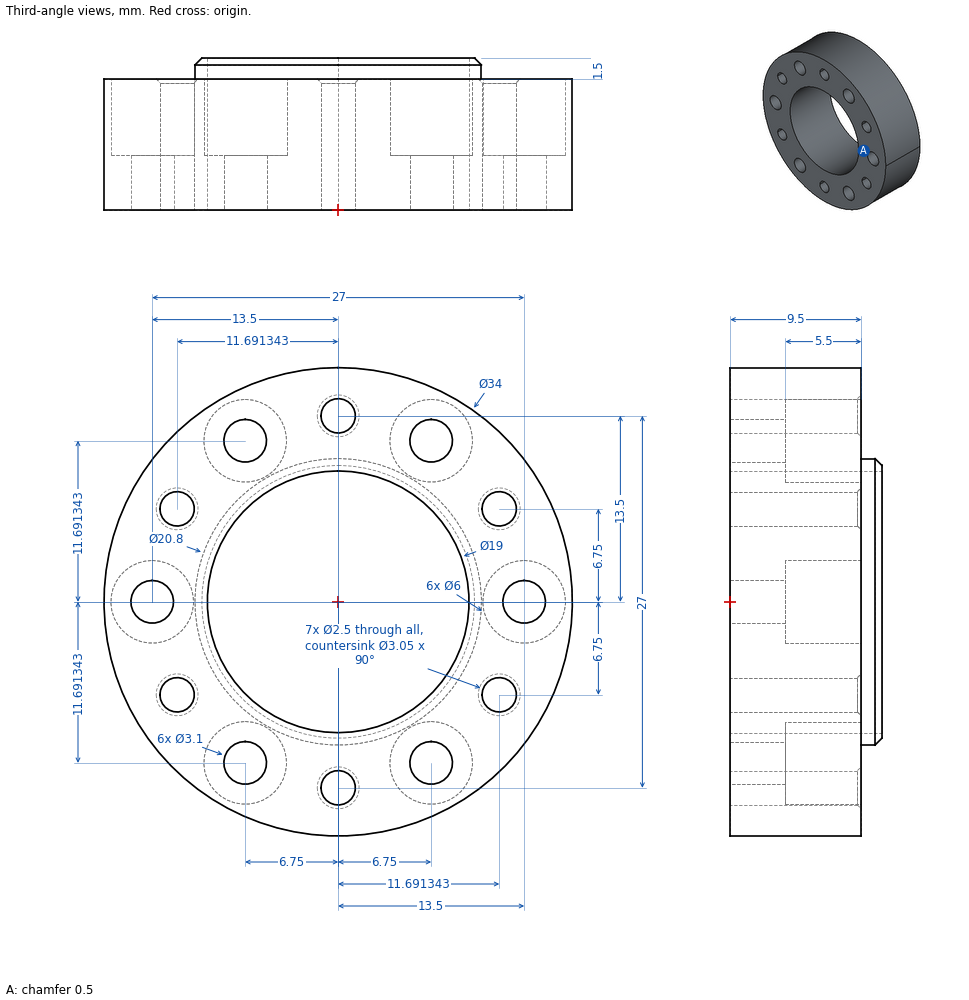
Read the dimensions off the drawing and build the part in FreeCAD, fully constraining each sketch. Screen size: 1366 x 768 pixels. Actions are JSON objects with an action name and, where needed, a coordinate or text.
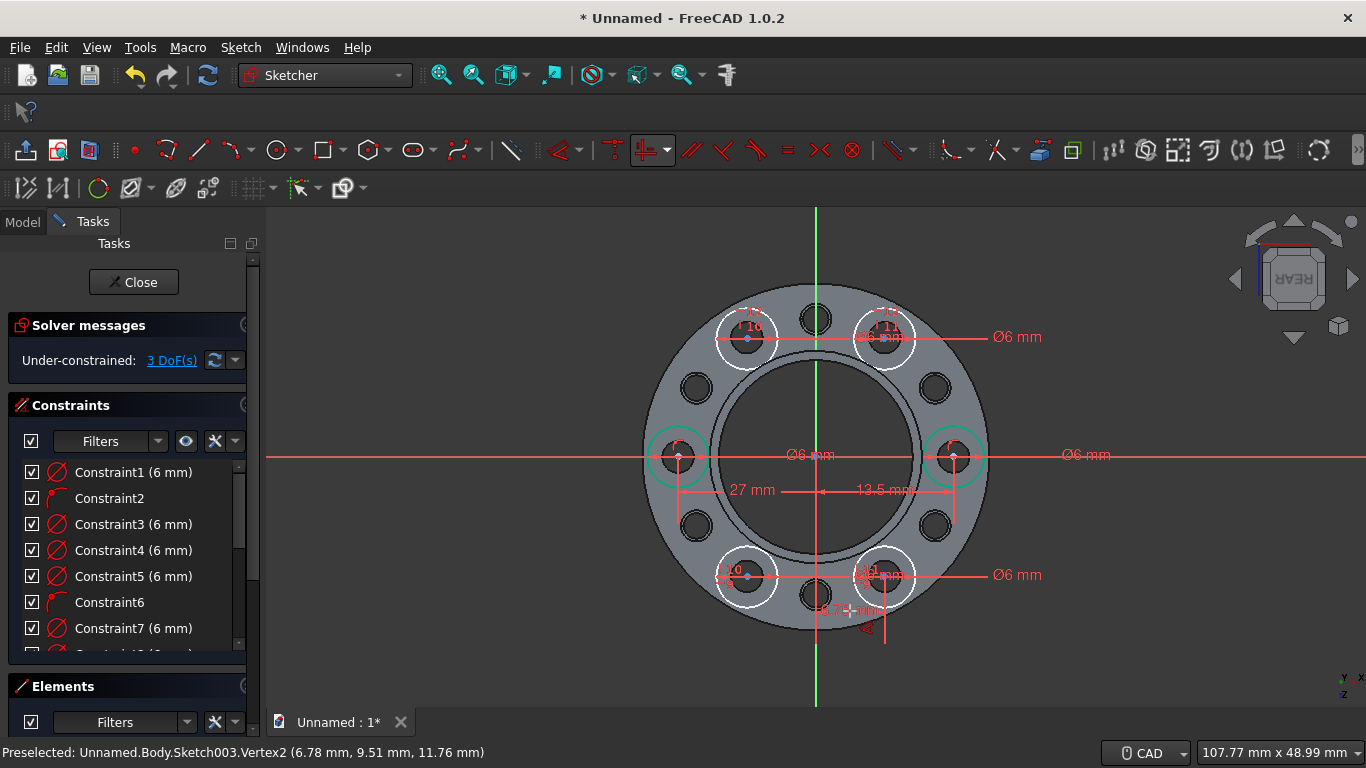
{"action": "left_click", "coordinate": [747, 577]}
{"action": "left_click", "coordinate": [781, 423]}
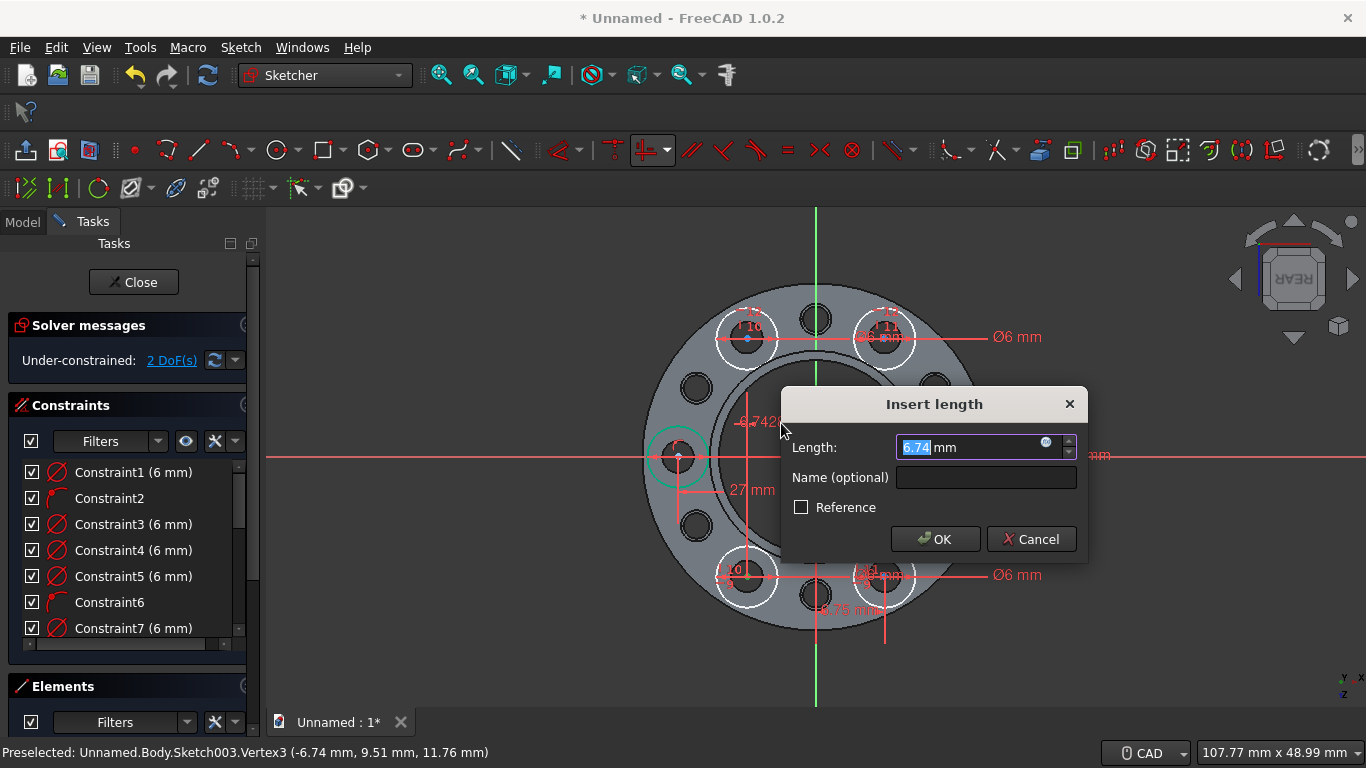
{"action": "type", "text": "6.75"}
{"action": "key", "text": "Return"}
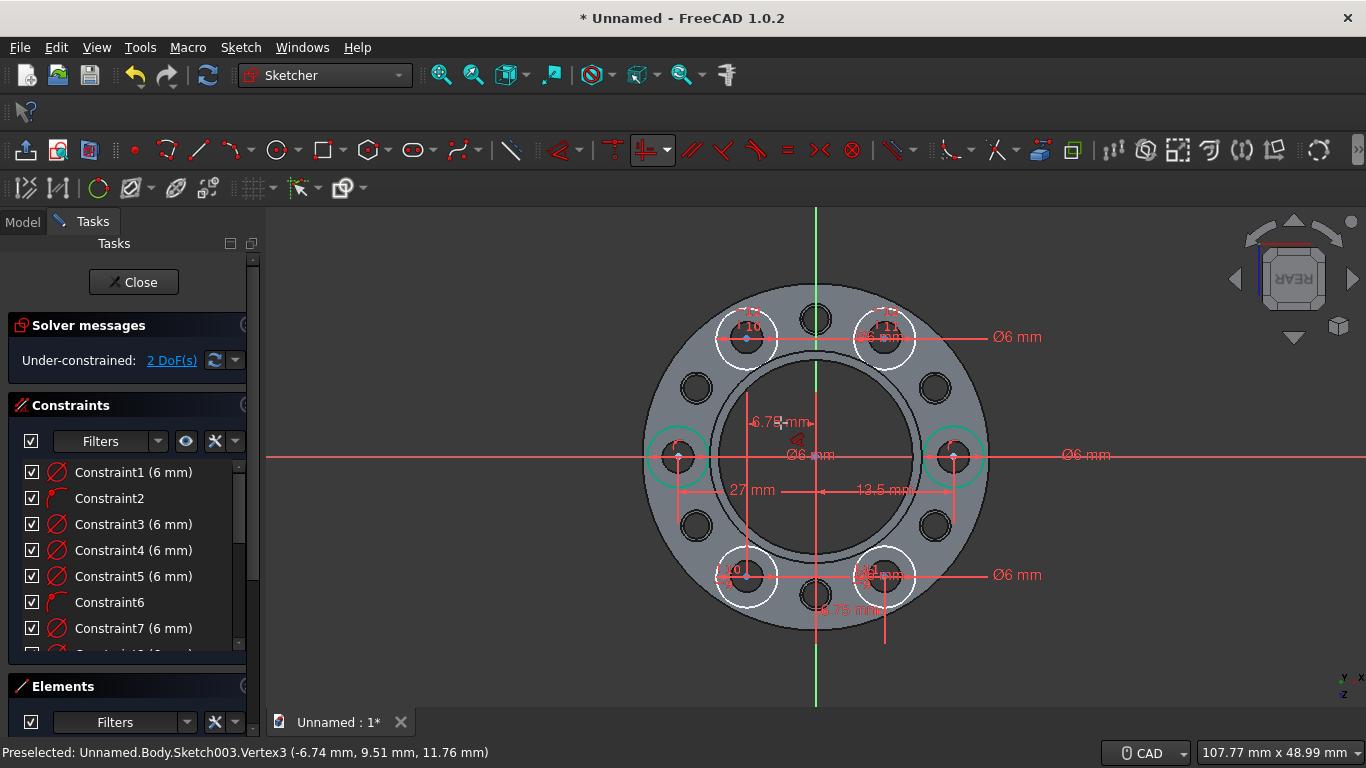
{"action": "left_click", "coordinate": [885, 577]}
{"action": "left_click", "coordinate": [919, 517]}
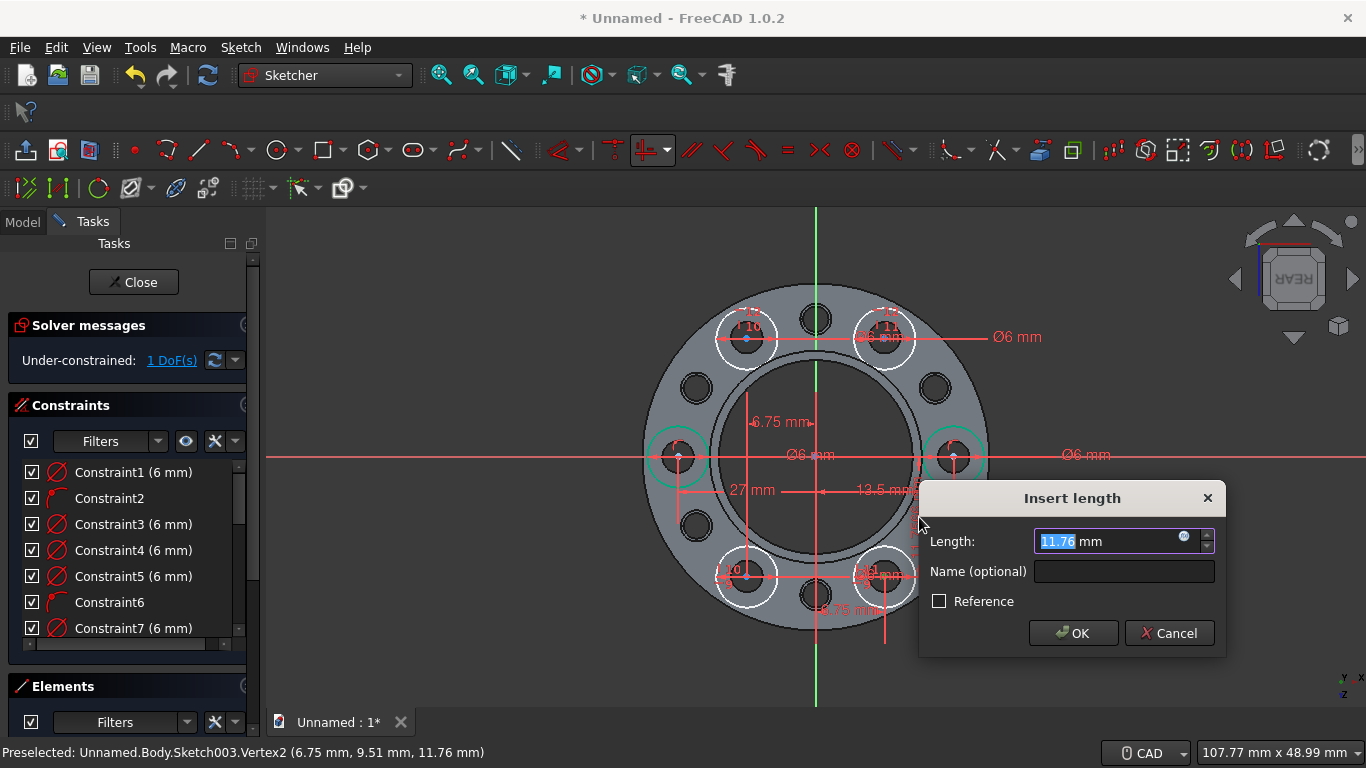
{"action": "type", "text": "11.691343"}
{"action": "key", "text": "Return"}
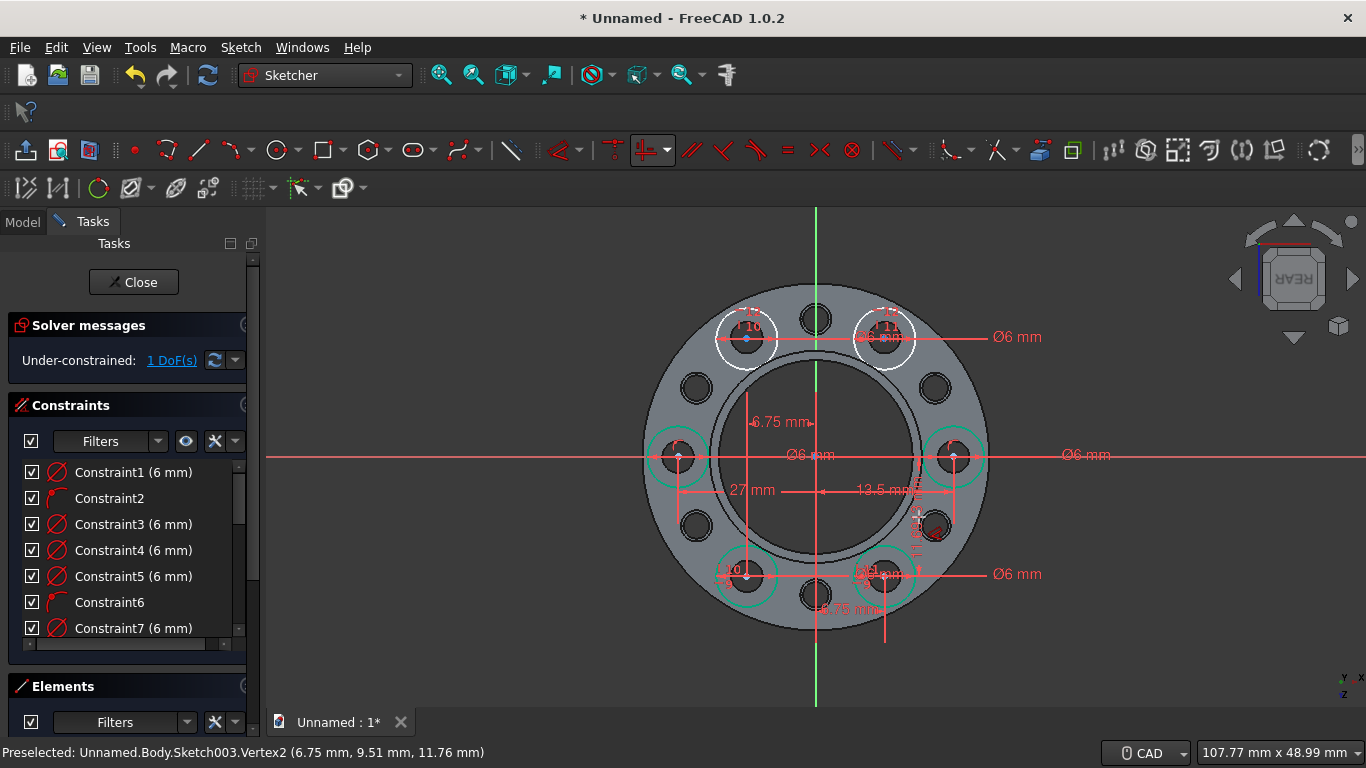
{"action": "left_click", "coordinate": [747, 339]}
{"action": "left_click", "coordinate": [713, 398]}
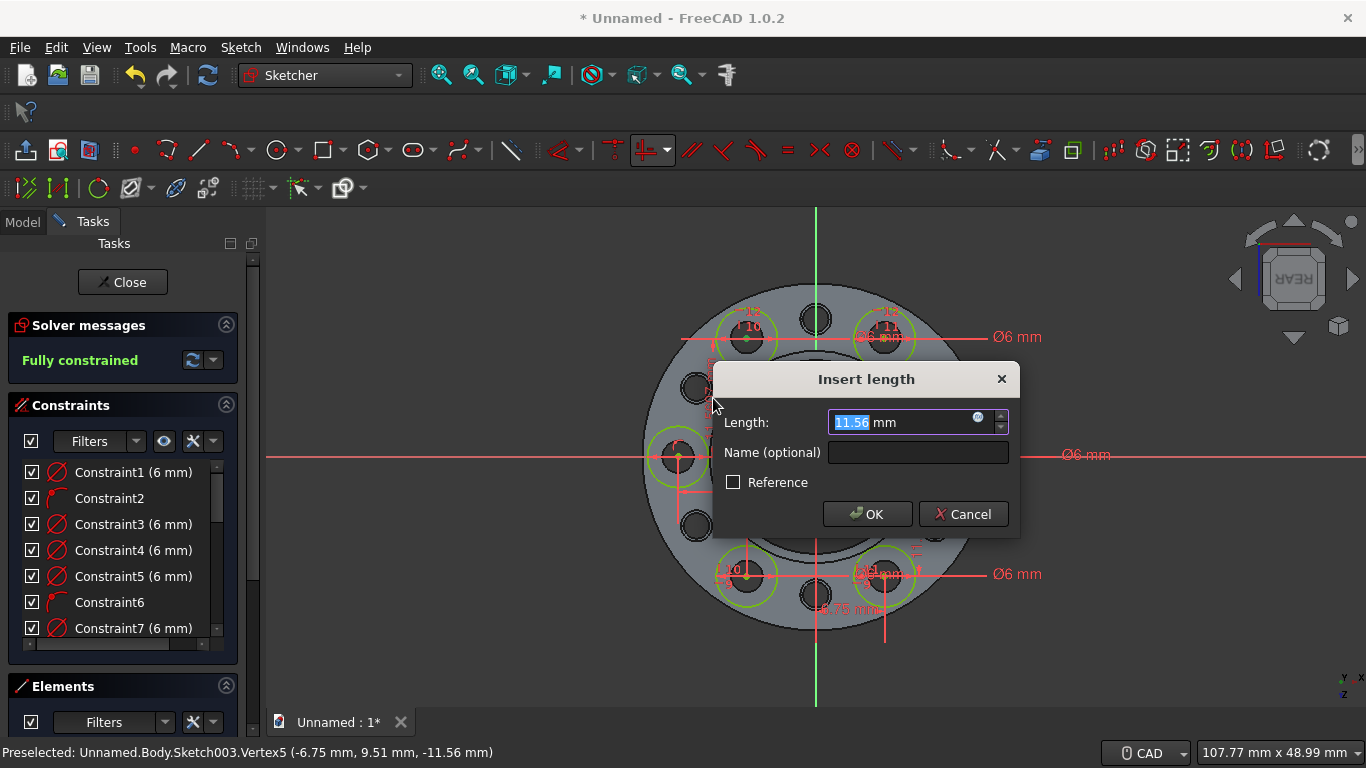
{"action": "type", "text": "11.691343"}
{"action": "key", "text": "Return"}
{"action": "key", "text": "Escape"}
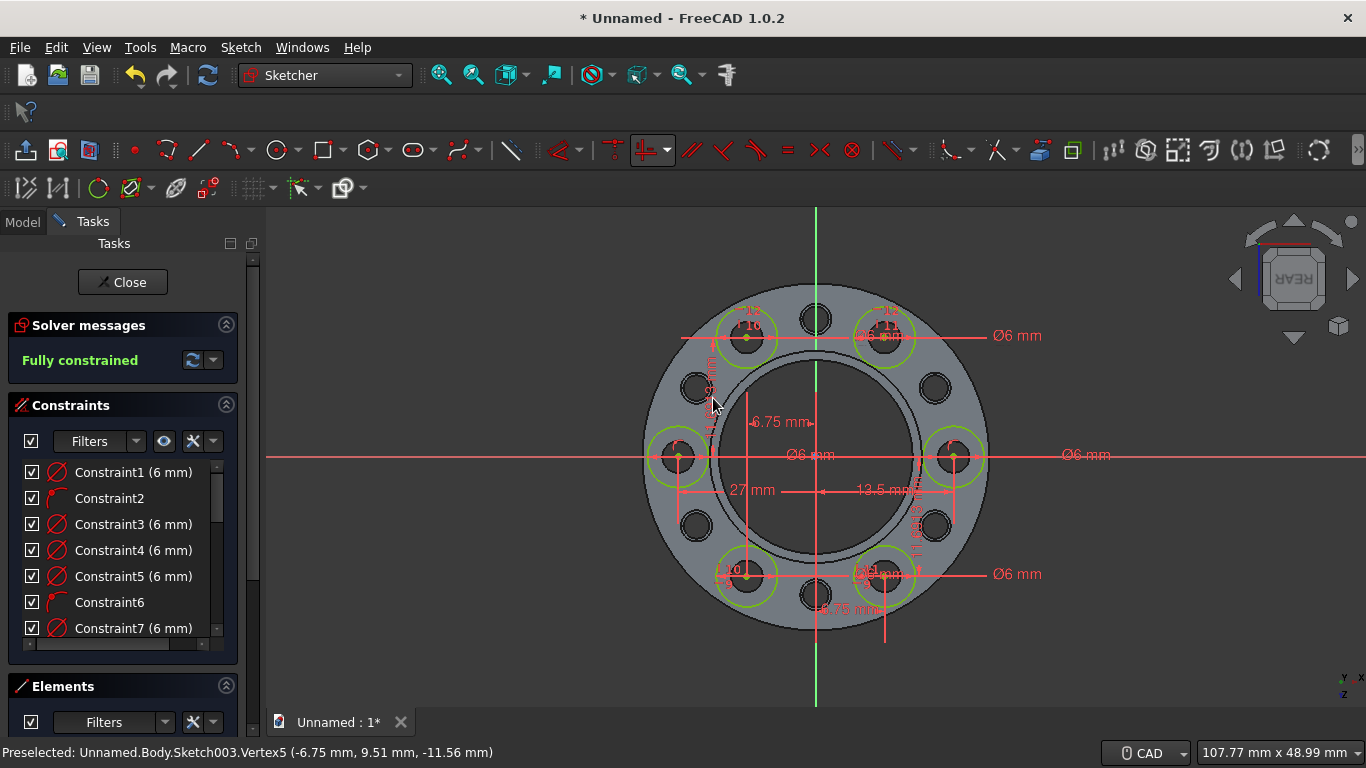
{"action": "left_click", "coordinate": [123, 282]}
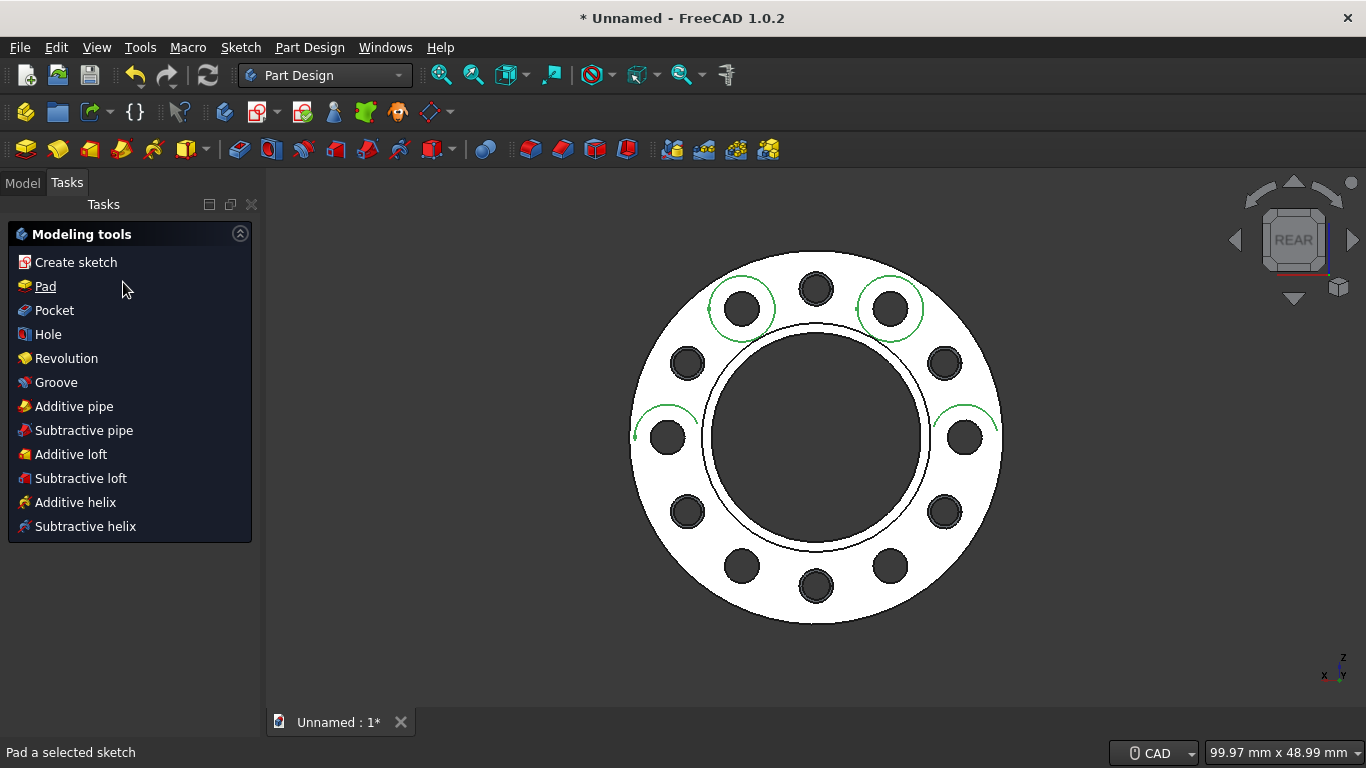
{"action": "left_click", "coordinate": [240, 150]}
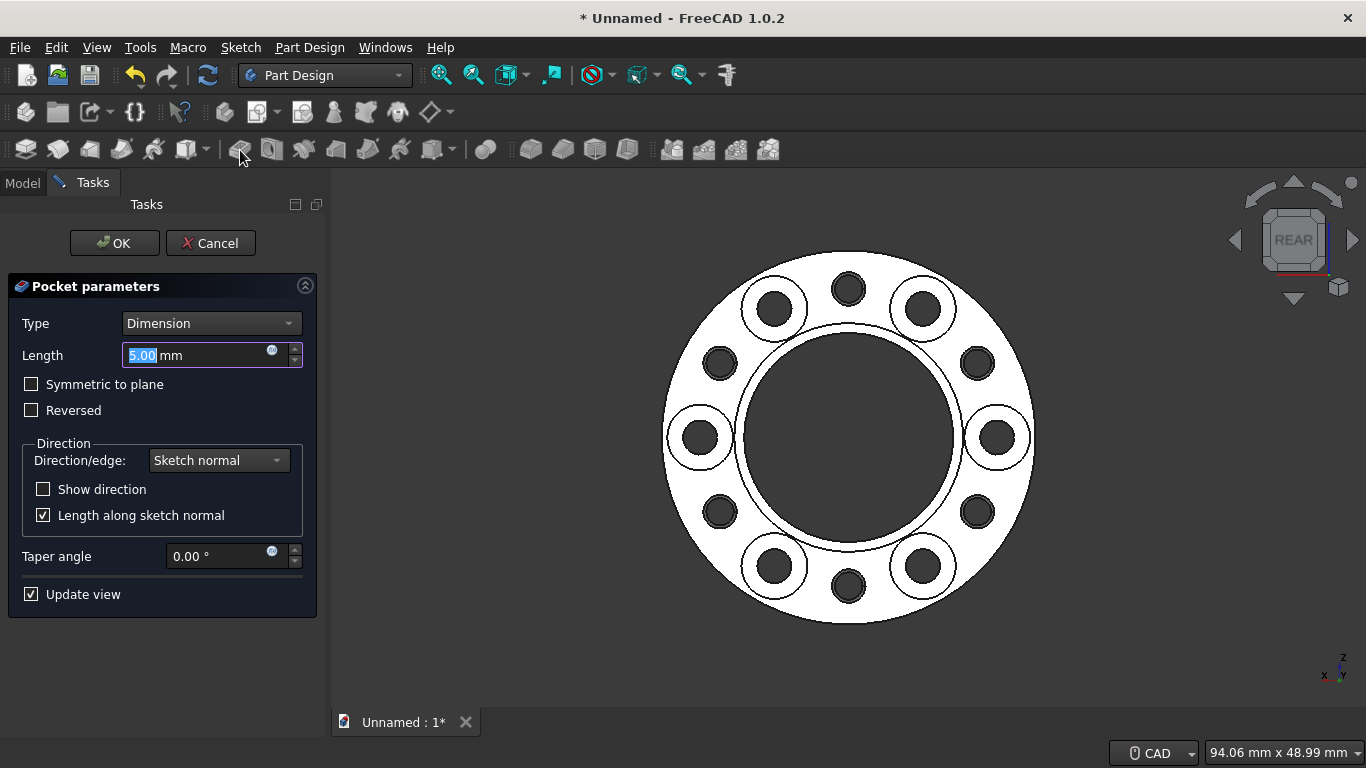
{"action": "type", "text": "5.5"}
{"action": "key", "text": "Tab"}